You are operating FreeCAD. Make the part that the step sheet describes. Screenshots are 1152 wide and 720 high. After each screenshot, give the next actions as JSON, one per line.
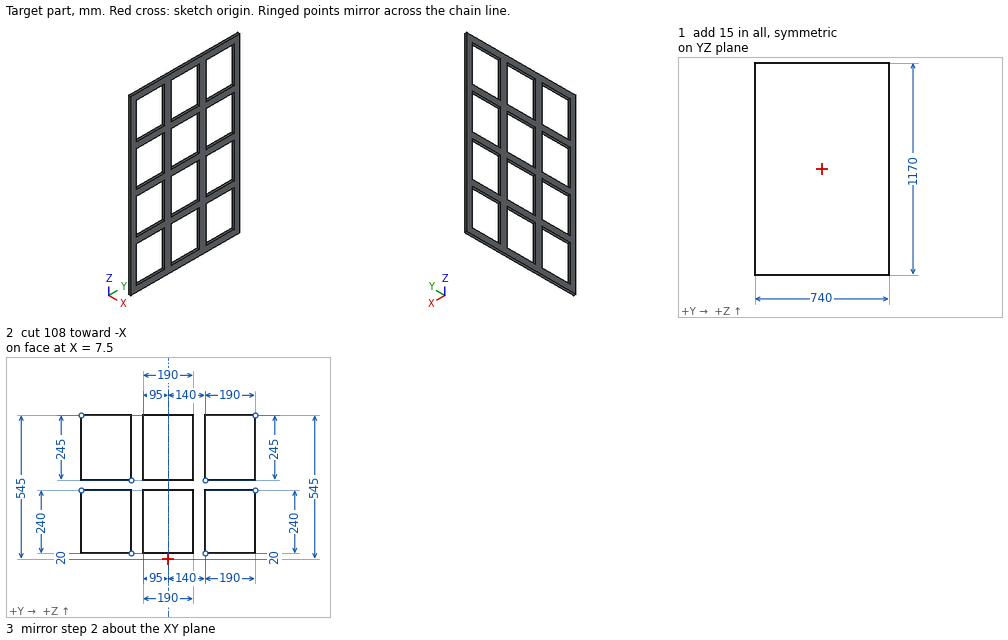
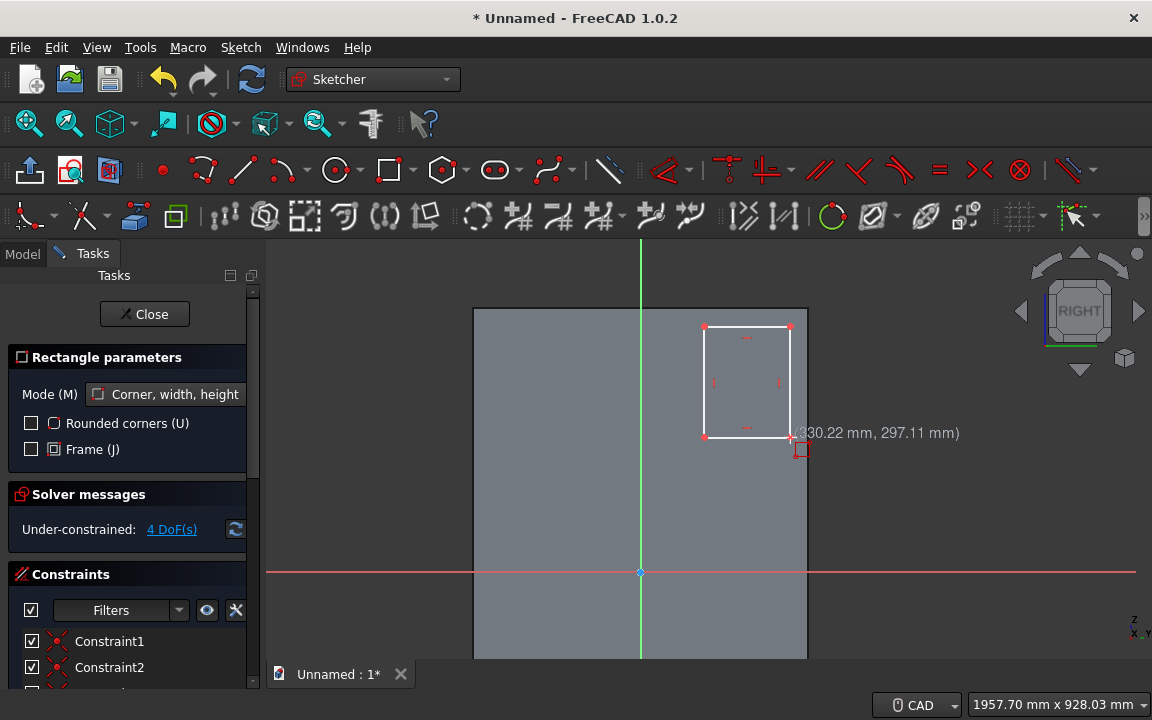
{"action": "left_click", "coordinate": [598, 326]}
{"action": "left_click", "coordinate": [684, 437]}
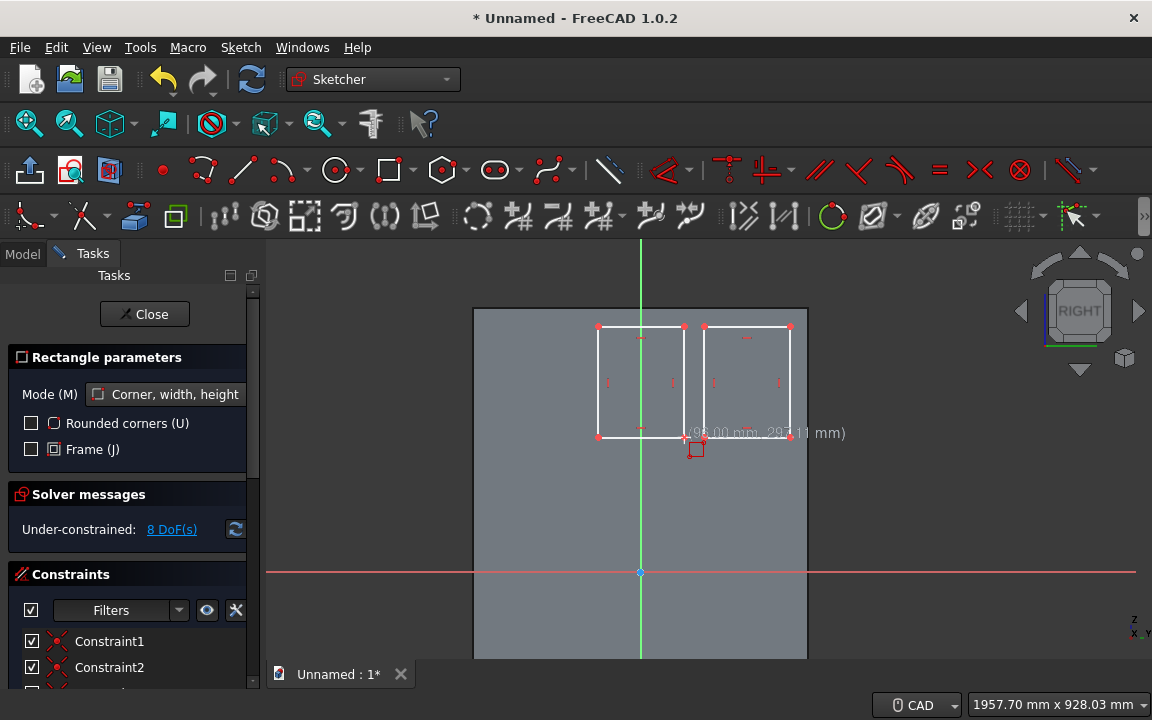
{"action": "left_click", "coordinate": [598, 455]}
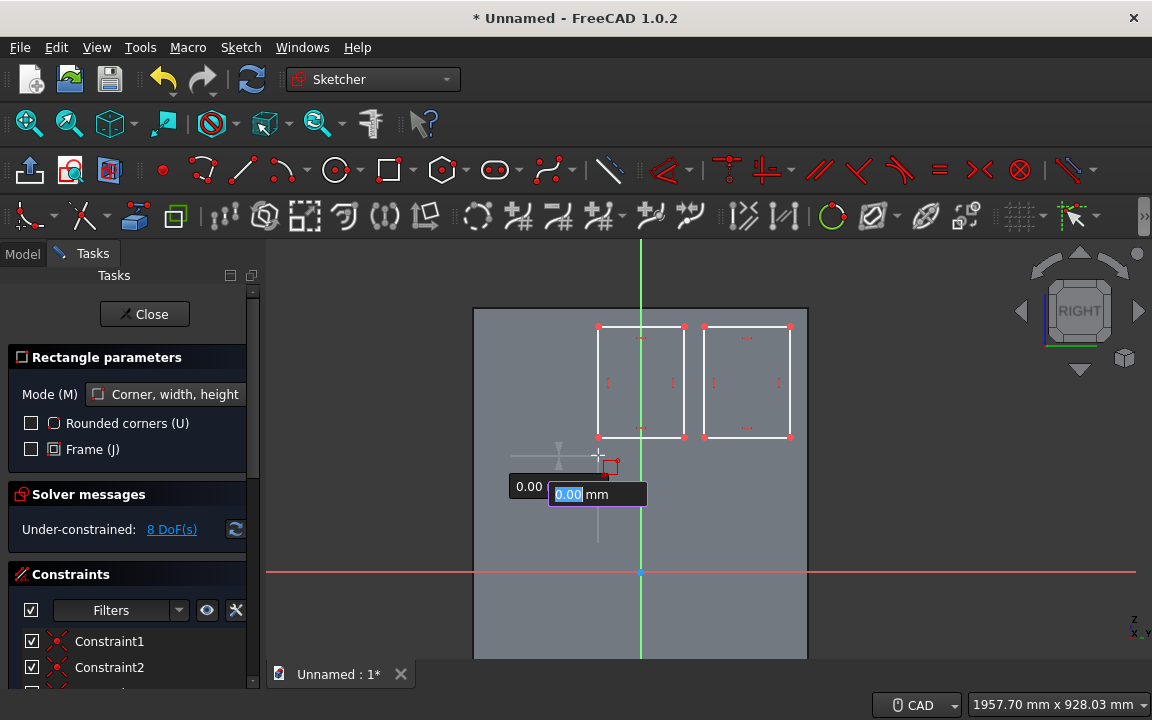
{"action": "scroll", "coordinate": [684, 563], "scroll_direction": "up", "scroll_amount": 3}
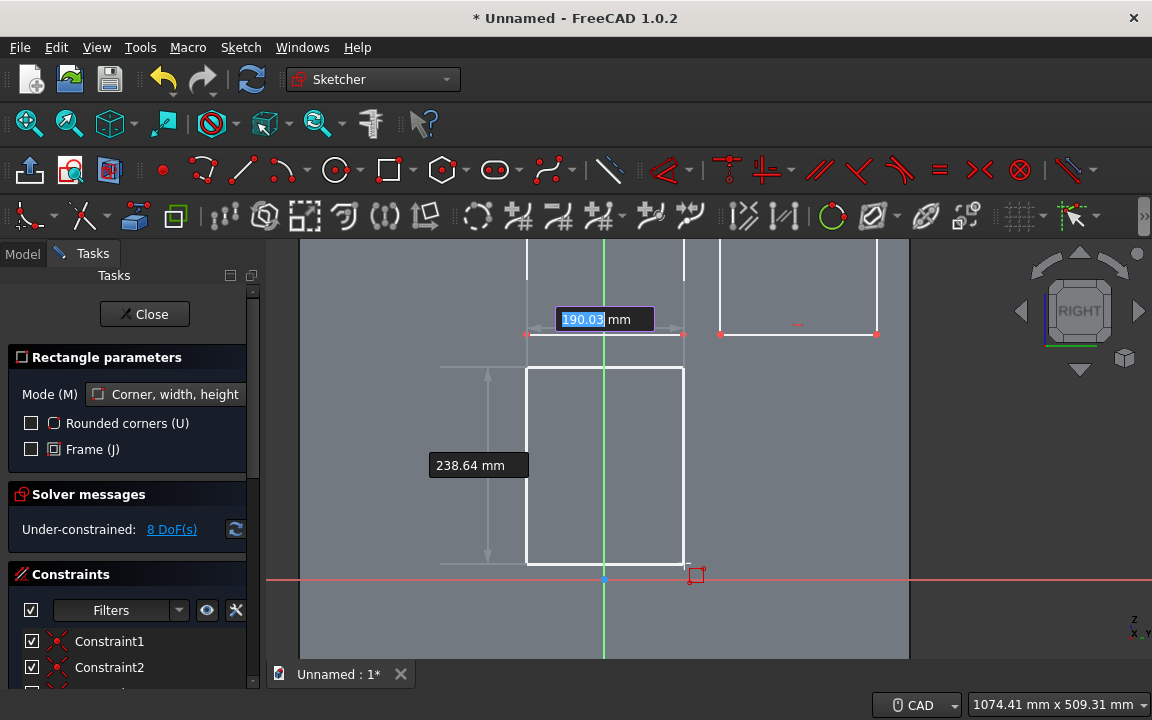
{"action": "left_click", "coordinate": [683, 563]}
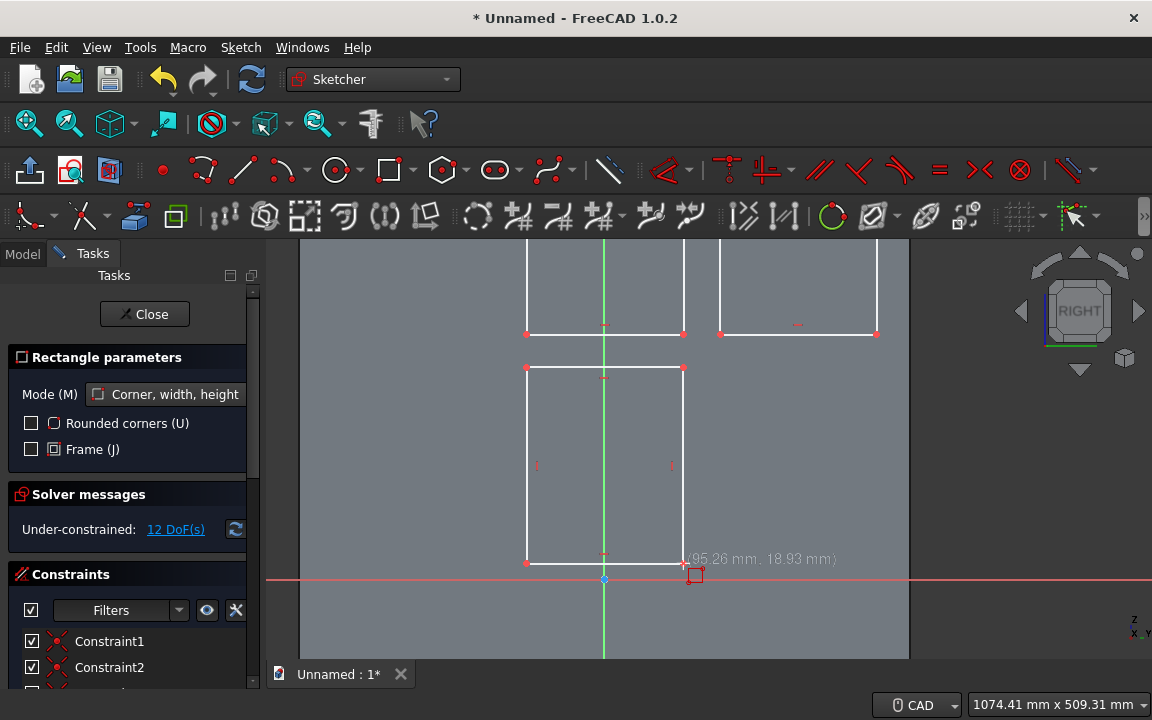
{"action": "left_click", "coordinate": [720, 365]}
{"action": "left_click", "coordinate": [877, 563]}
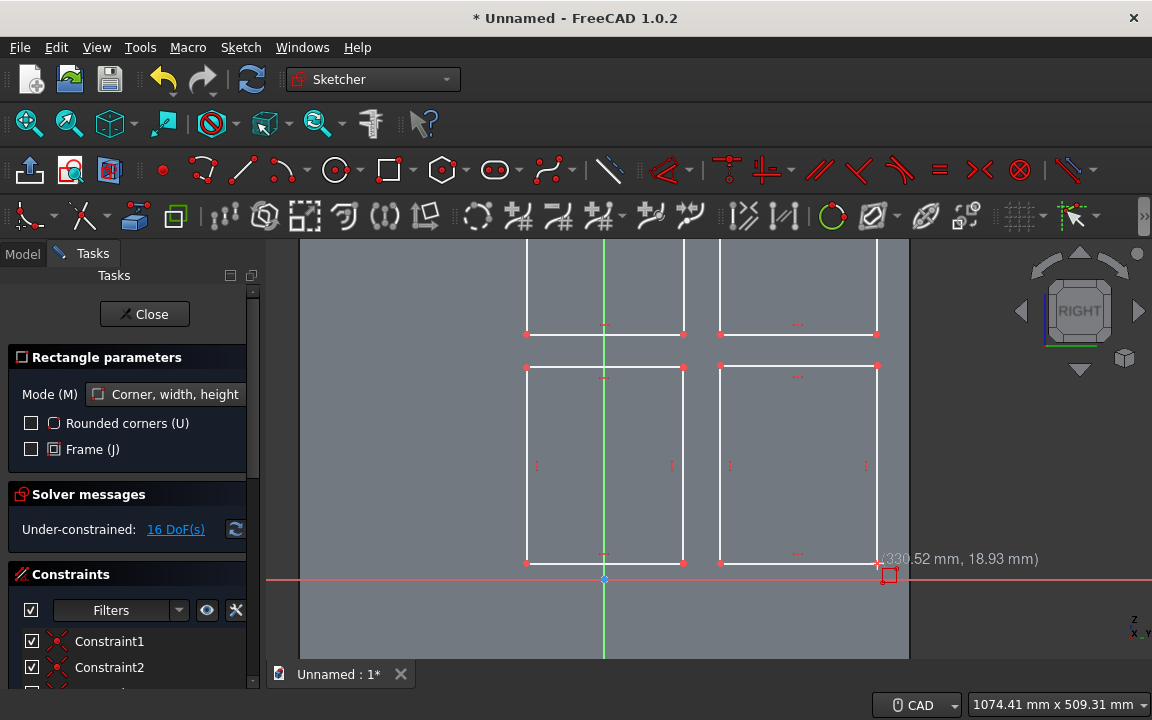
{"action": "scroll", "coordinate": [684, 563], "scroll_direction": "down", "scroll_amount": 3}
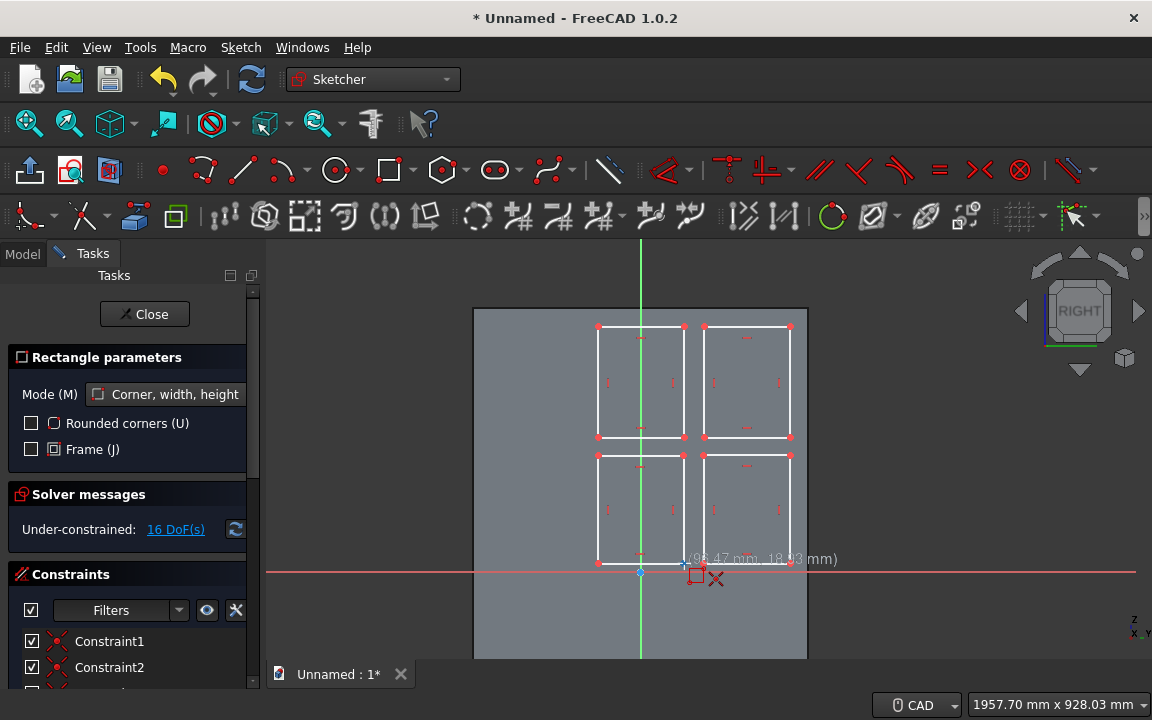
{"action": "left_click", "coordinate": [491, 326]}
{"action": "left_click", "coordinate": [577, 437]}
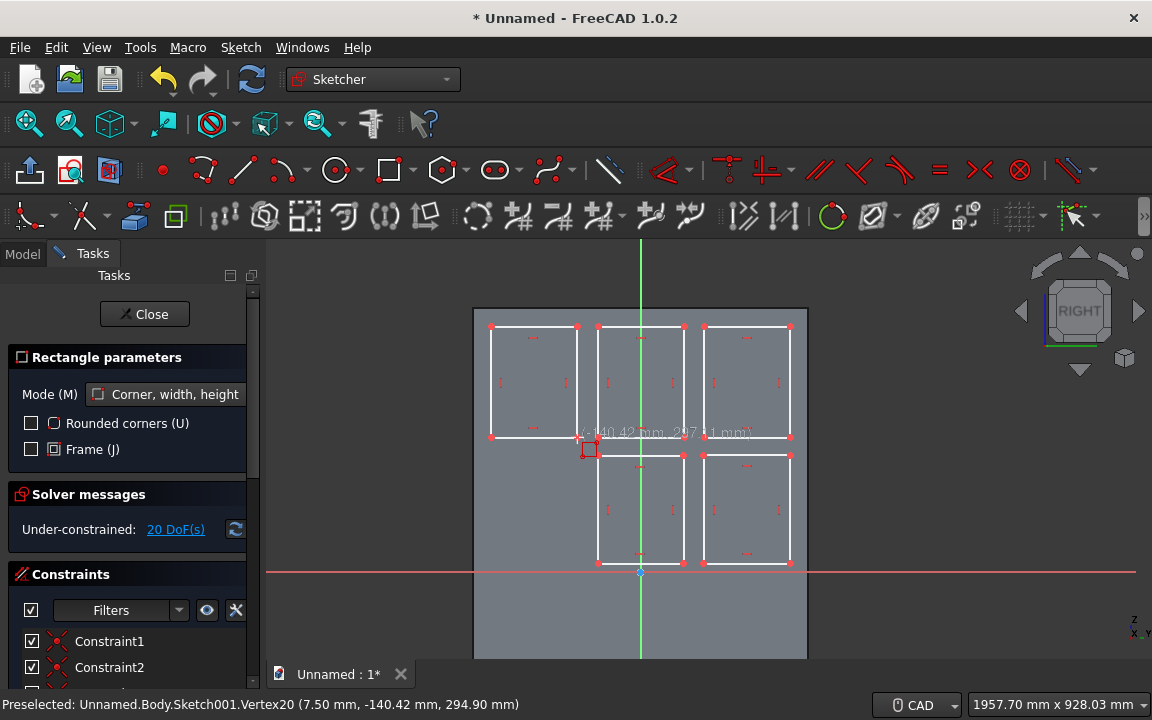
{"action": "left_click", "coordinate": [491, 455]}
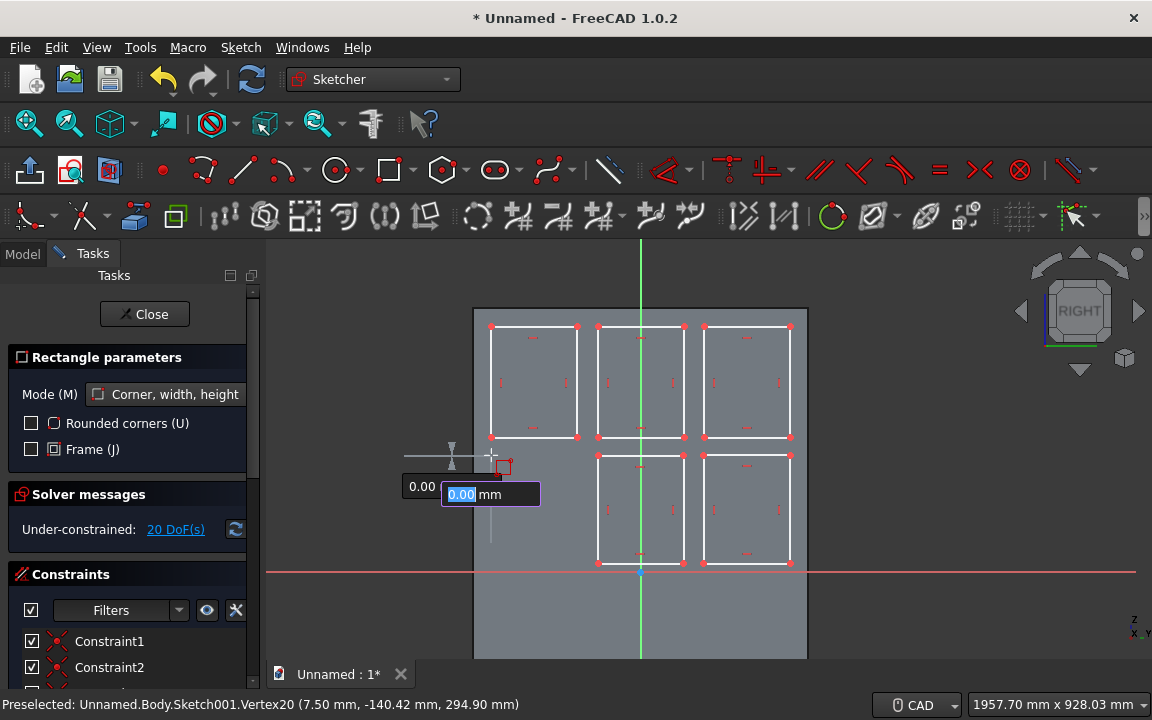
{"action": "scroll", "coordinate": [577, 563], "scroll_direction": "up", "scroll_amount": 3}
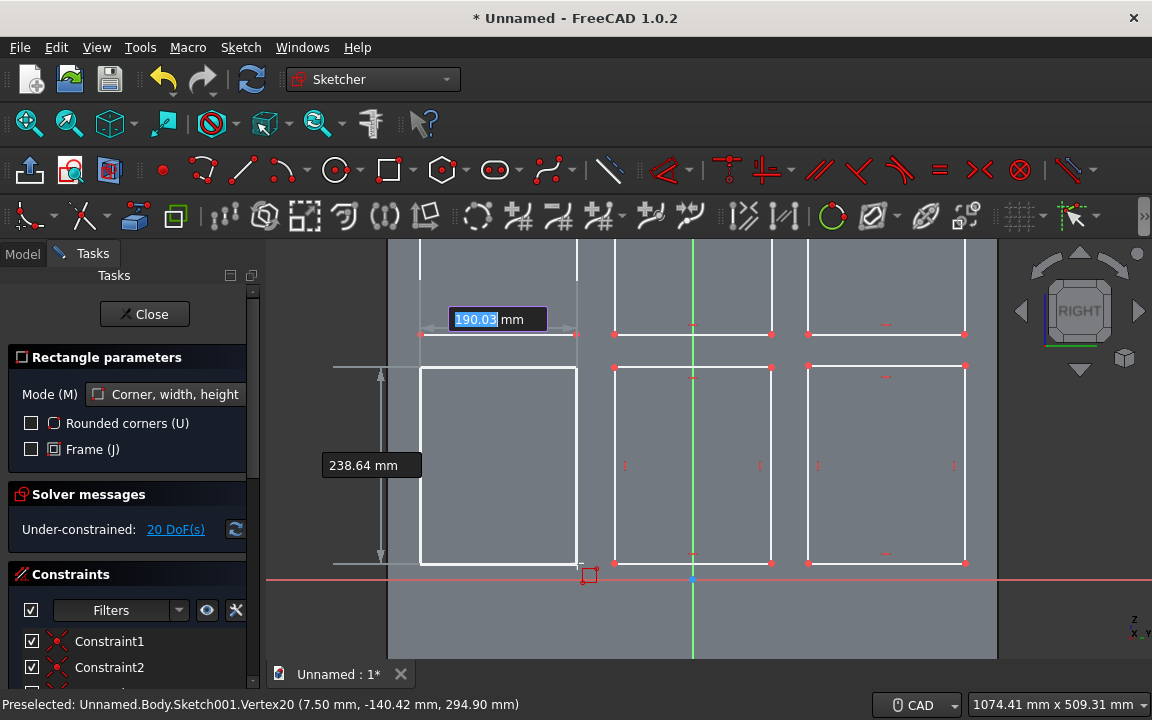
{"action": "left_click", "coordinate": [577, 563]}
{"action": "key", "text": "Escape"}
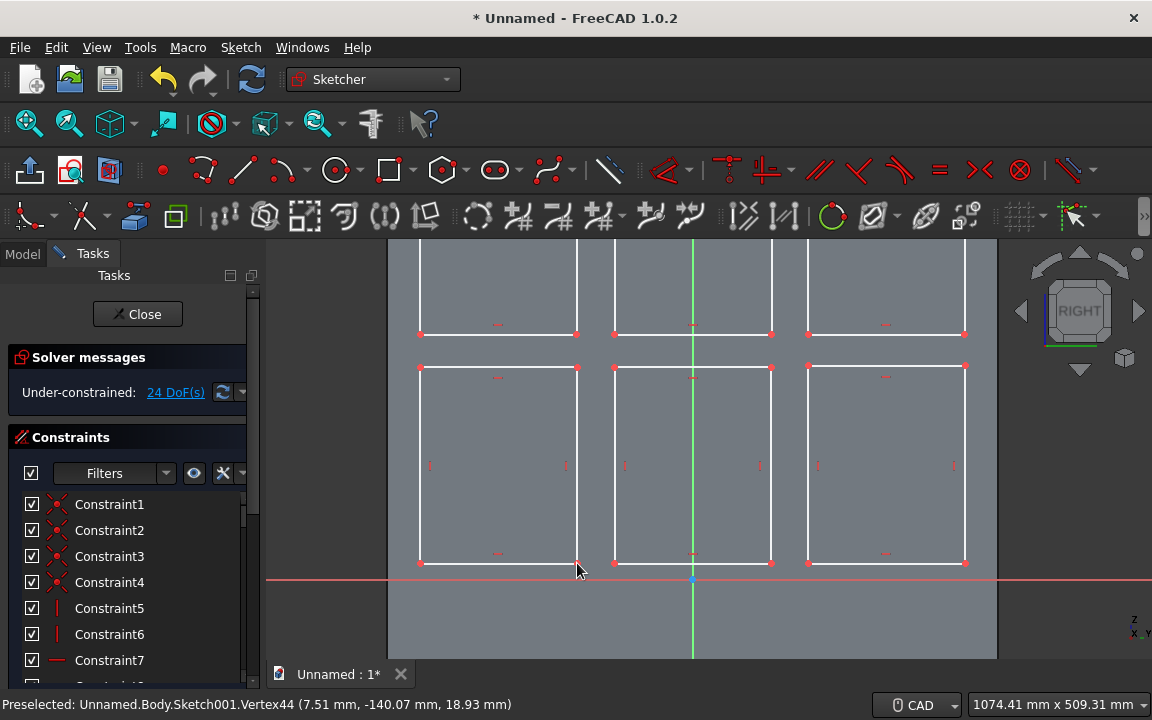
{"action": "scroll", "coordinate": [577, 563], "scroll_direction": "down", "scroll_amount": 3}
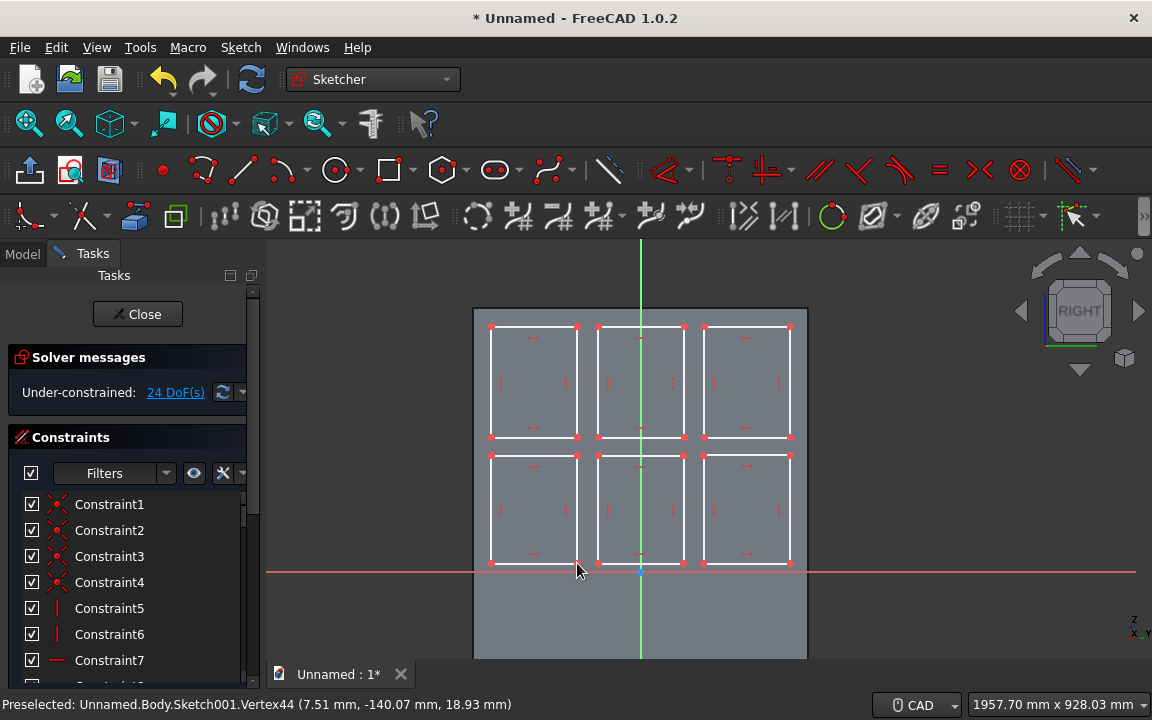
{"action": "left_click", "coordinate": [790, 327]}